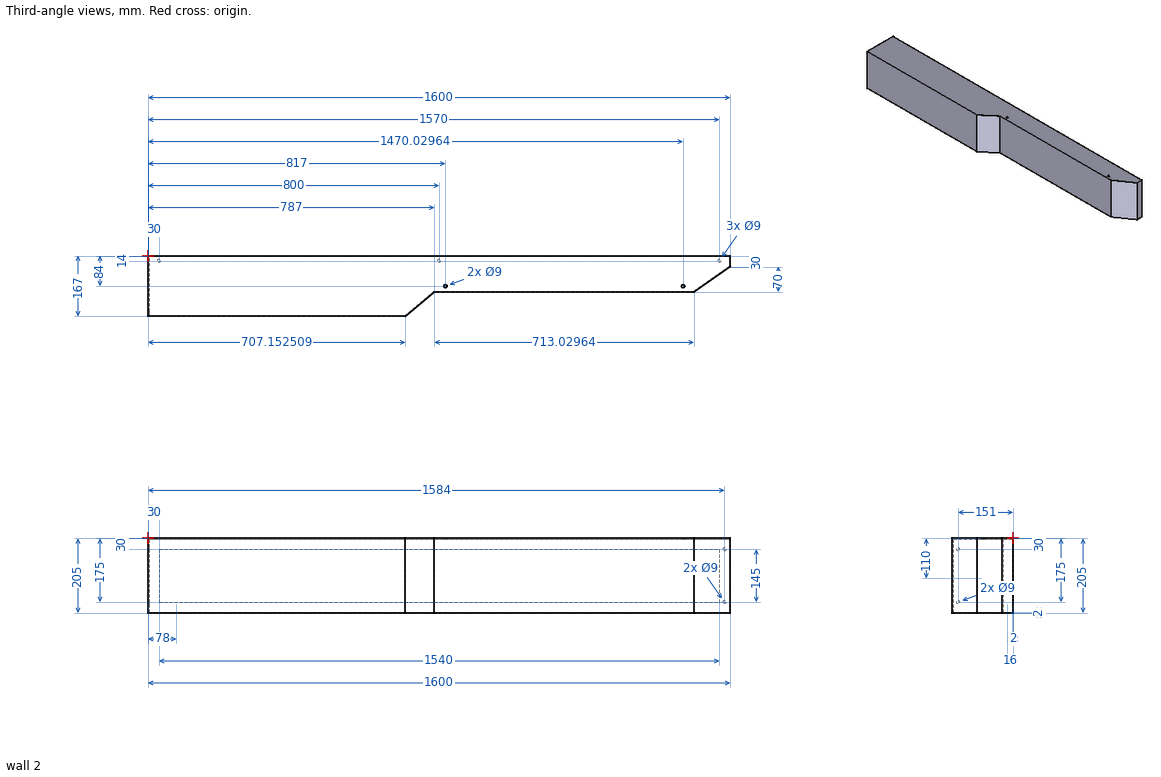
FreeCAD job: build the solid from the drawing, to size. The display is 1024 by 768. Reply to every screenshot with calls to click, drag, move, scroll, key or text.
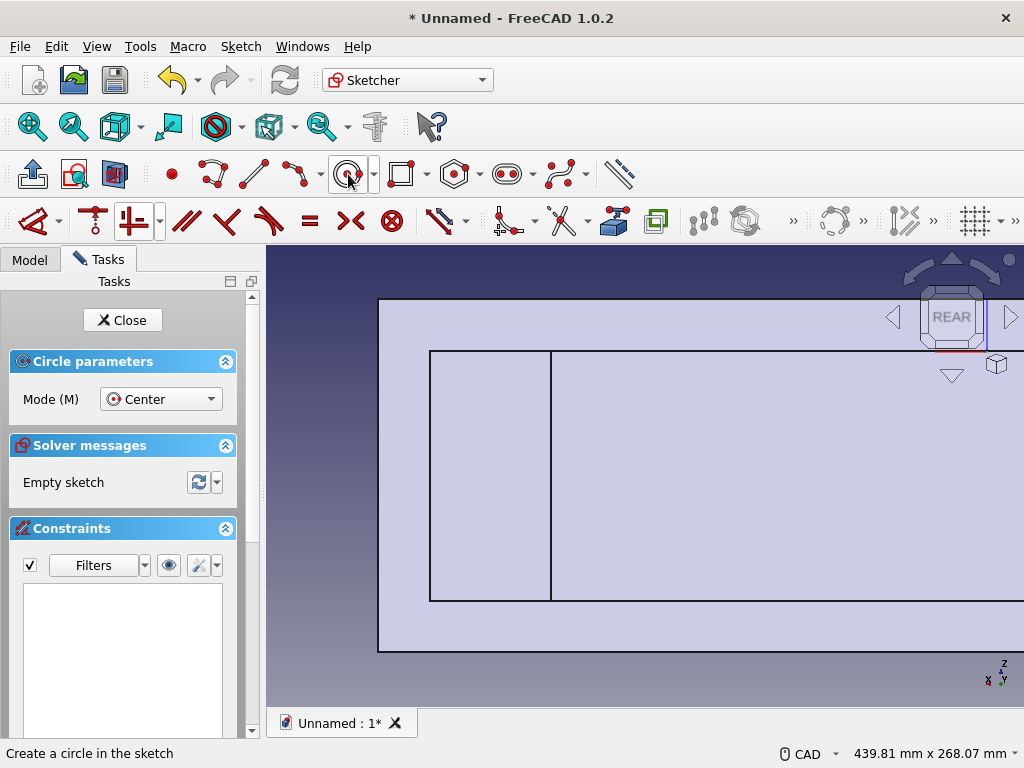
scroll(406, 601, up, 6)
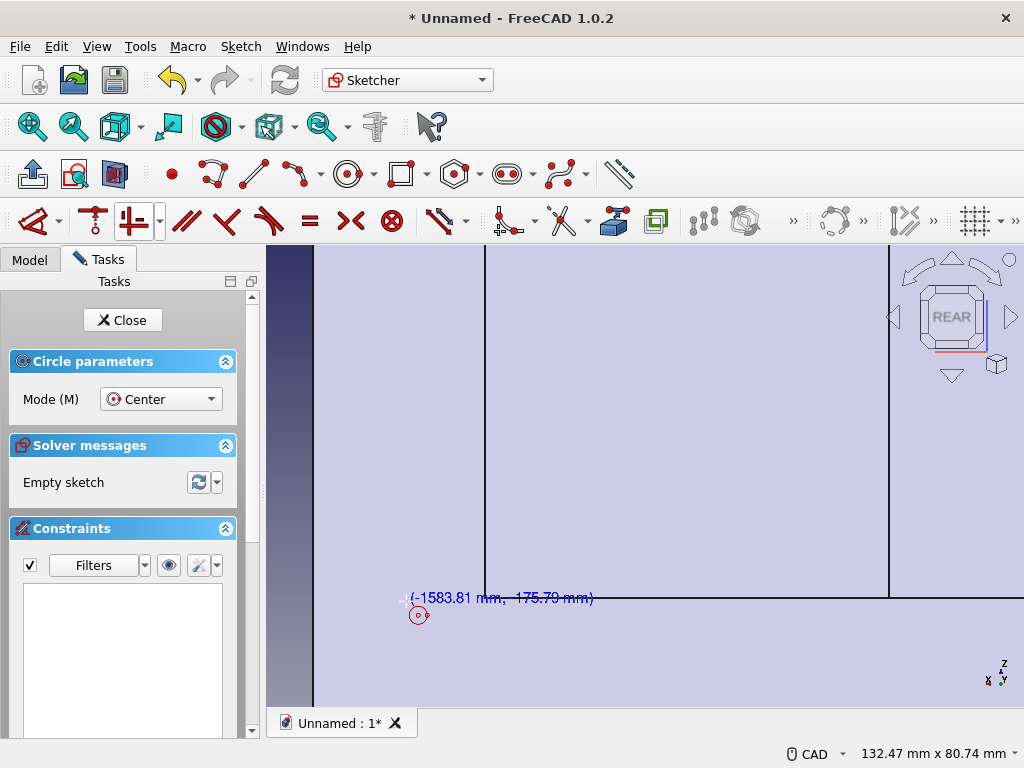
click(405, 598)
move(423, 580)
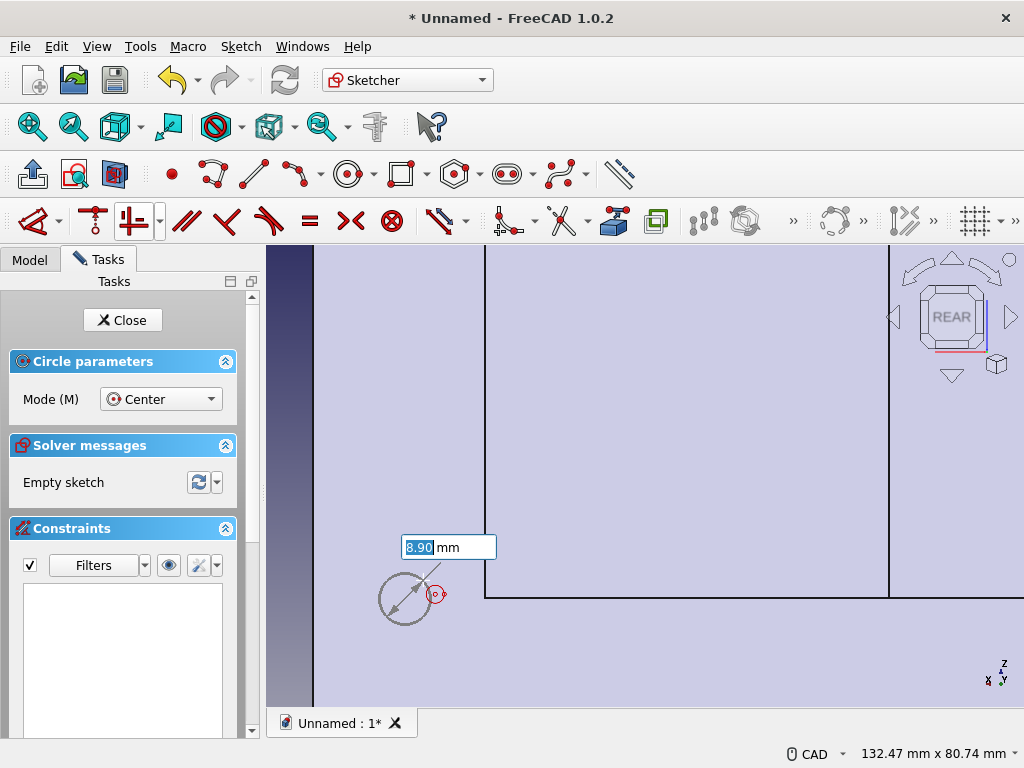
text(9)
key(Return)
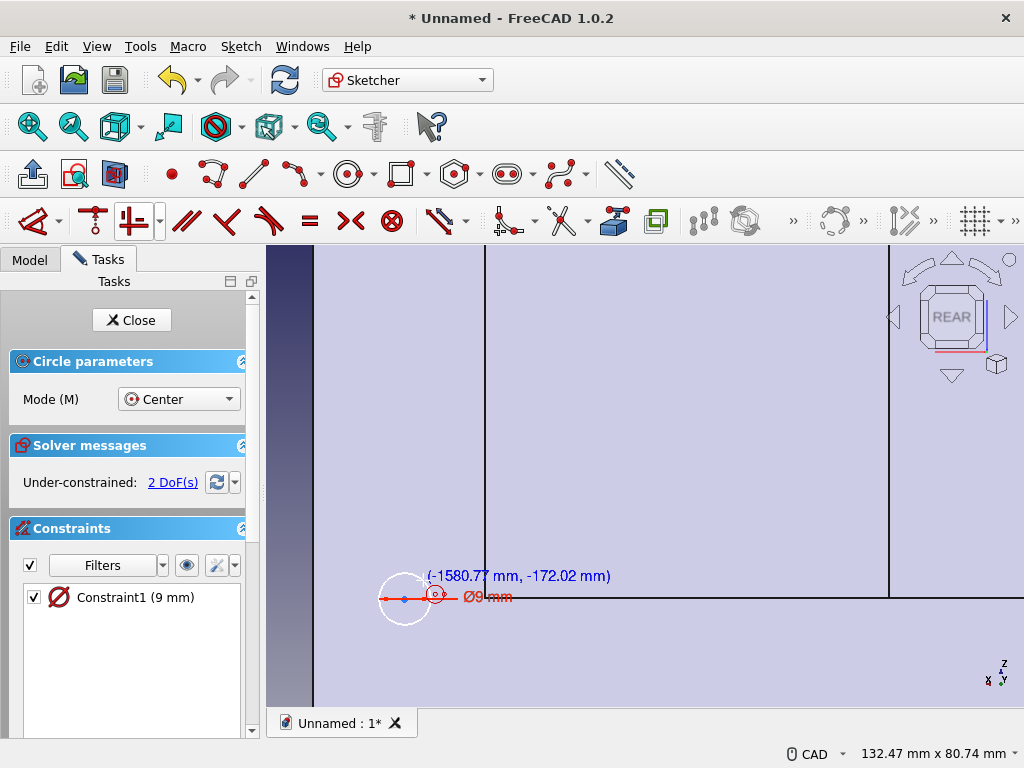
scroll(651, 602, down, 6)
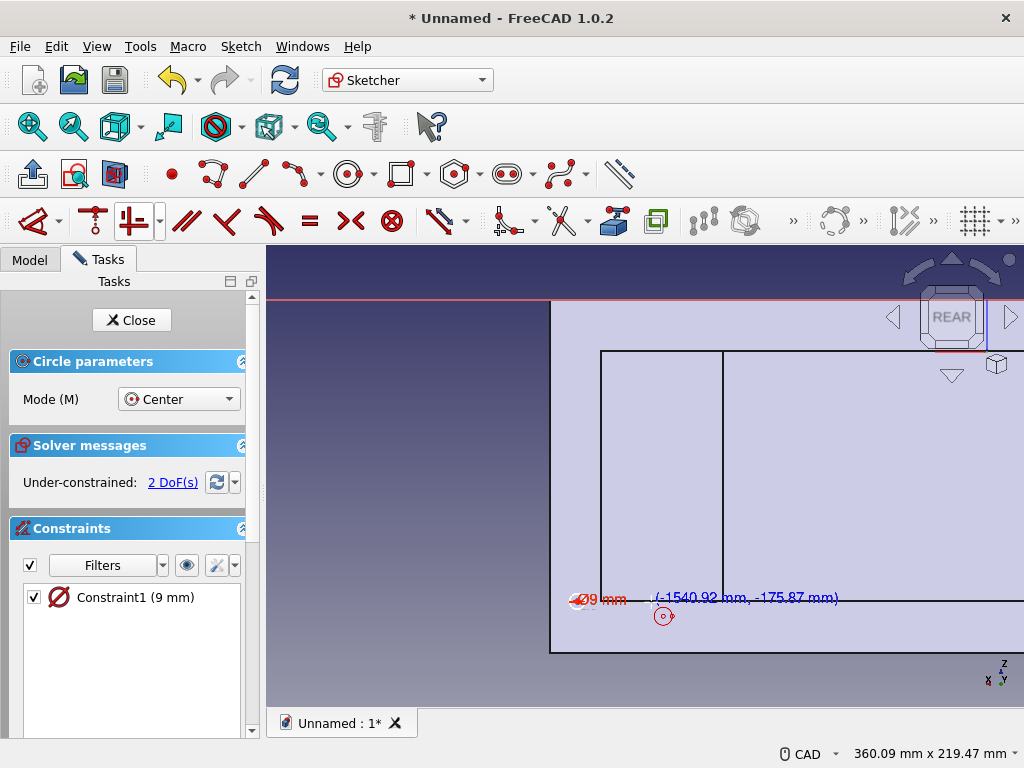
scroll(577, 351, up, 6)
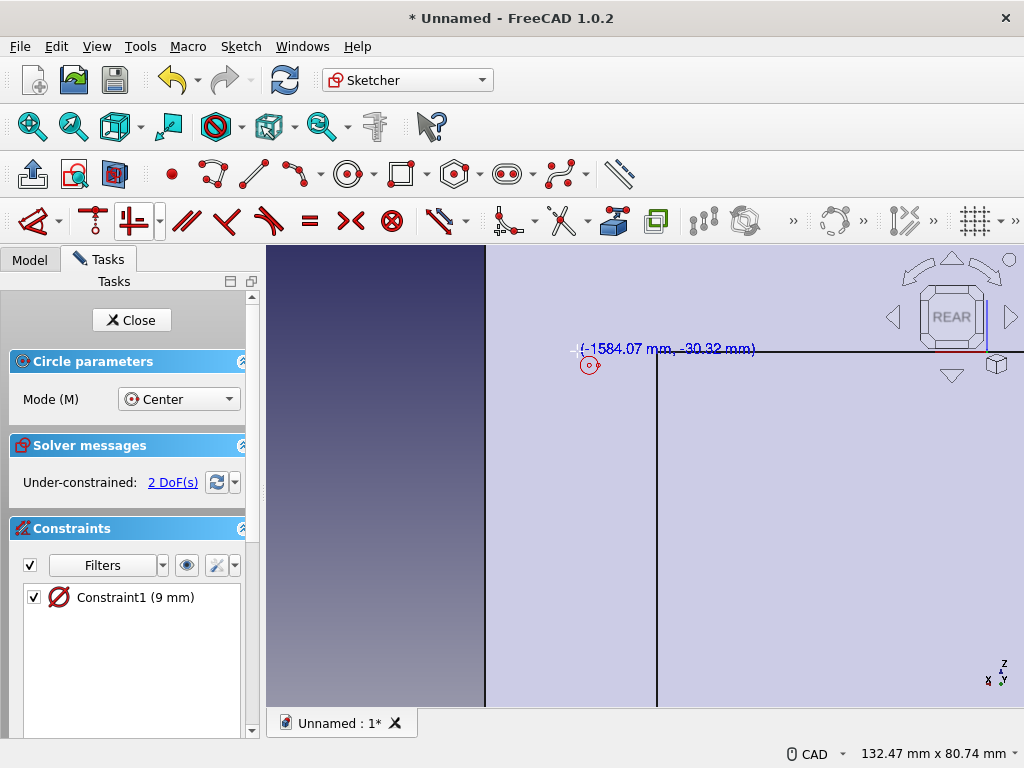
click(576, 352)
move(595, 334)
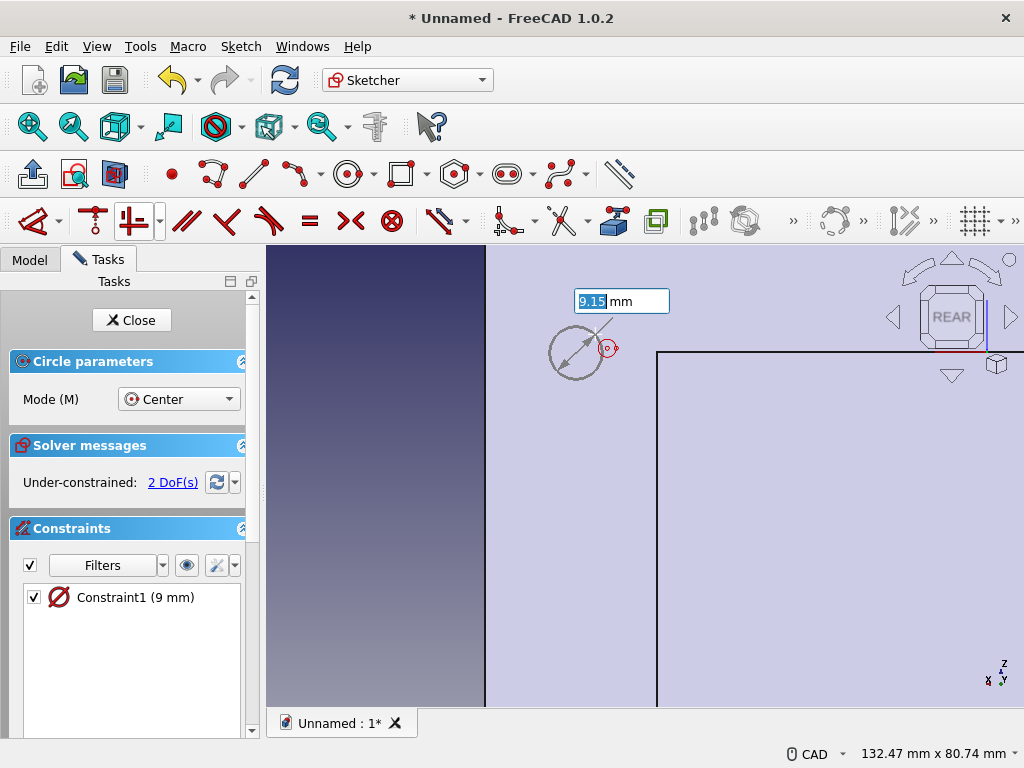
text(9)
key(Return)
key(Escape)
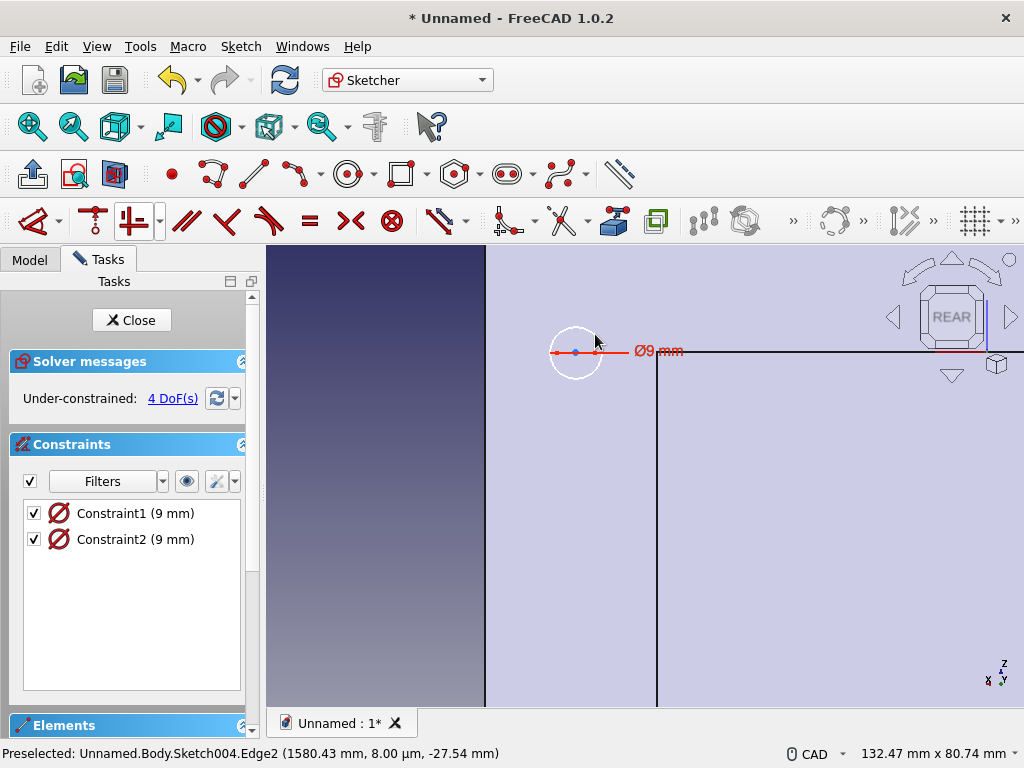
key(d)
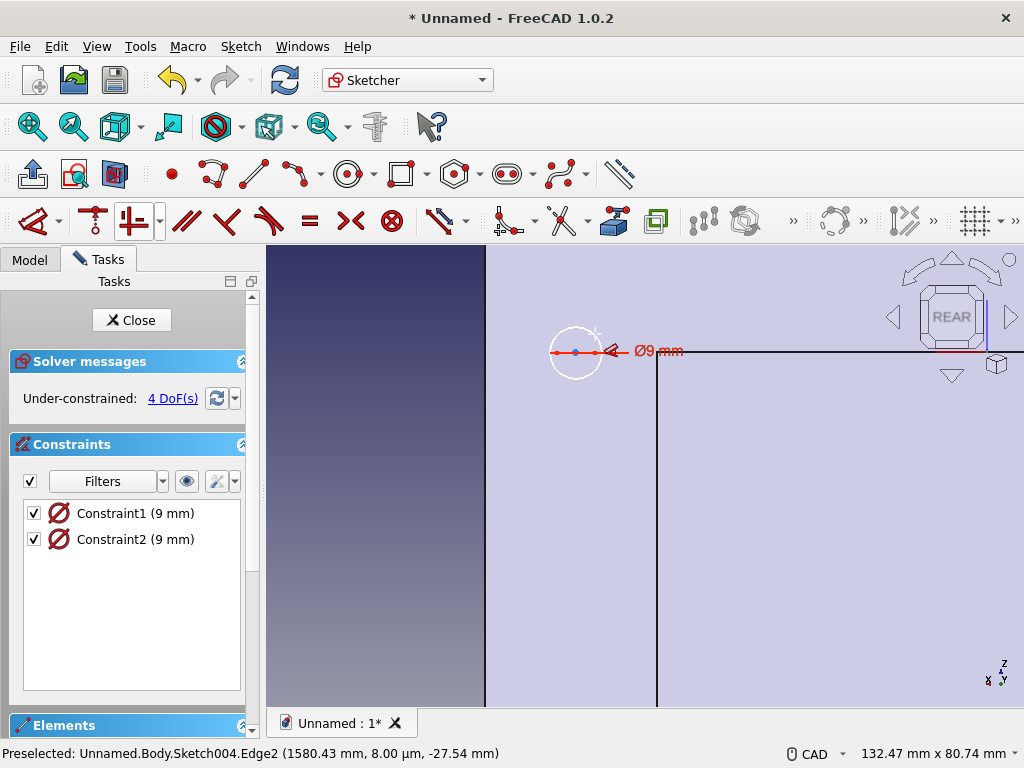
click(576, 353)
click(542, 313)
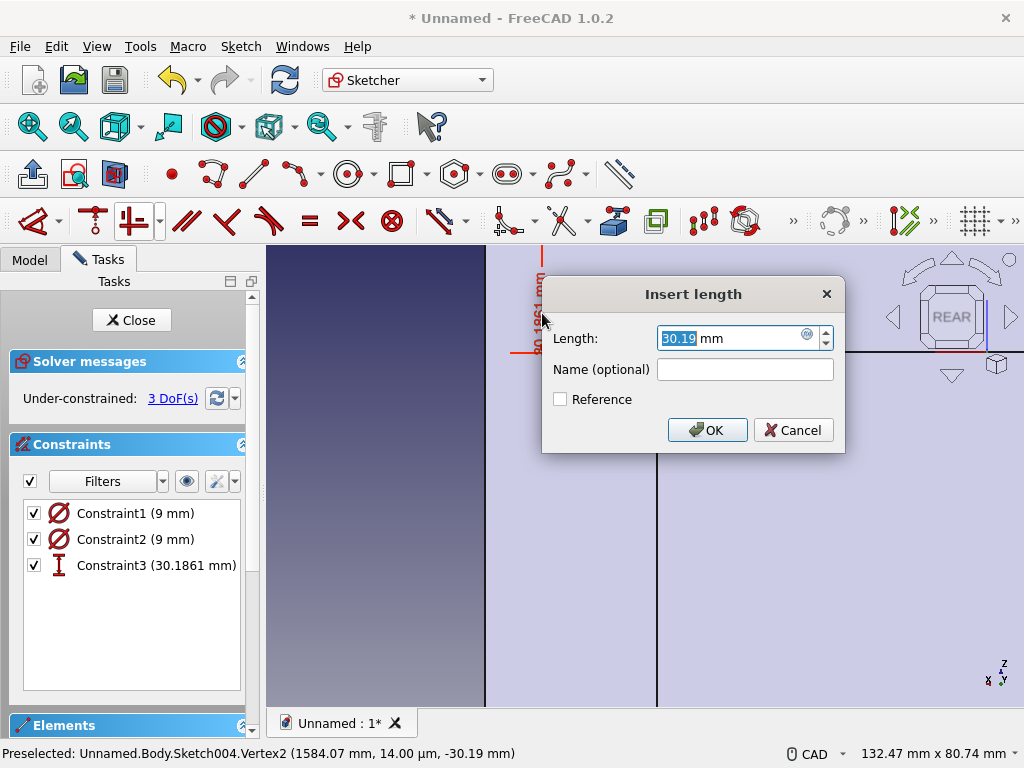
text(30)
key(Return)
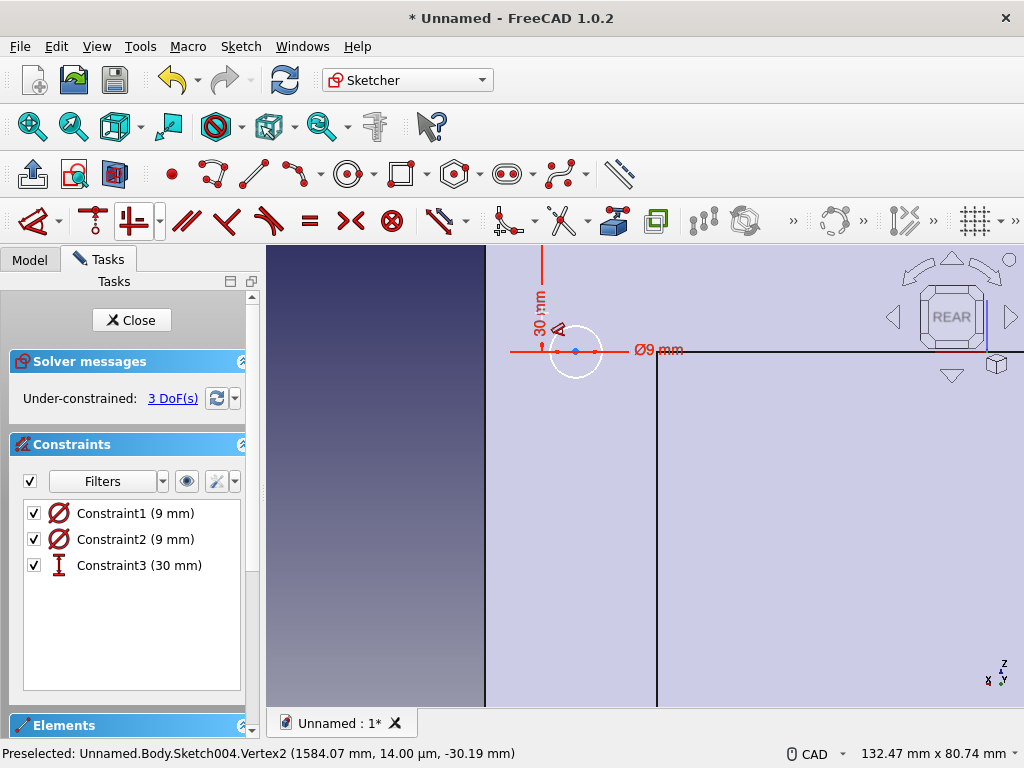
scroll(577, 351, down, 6)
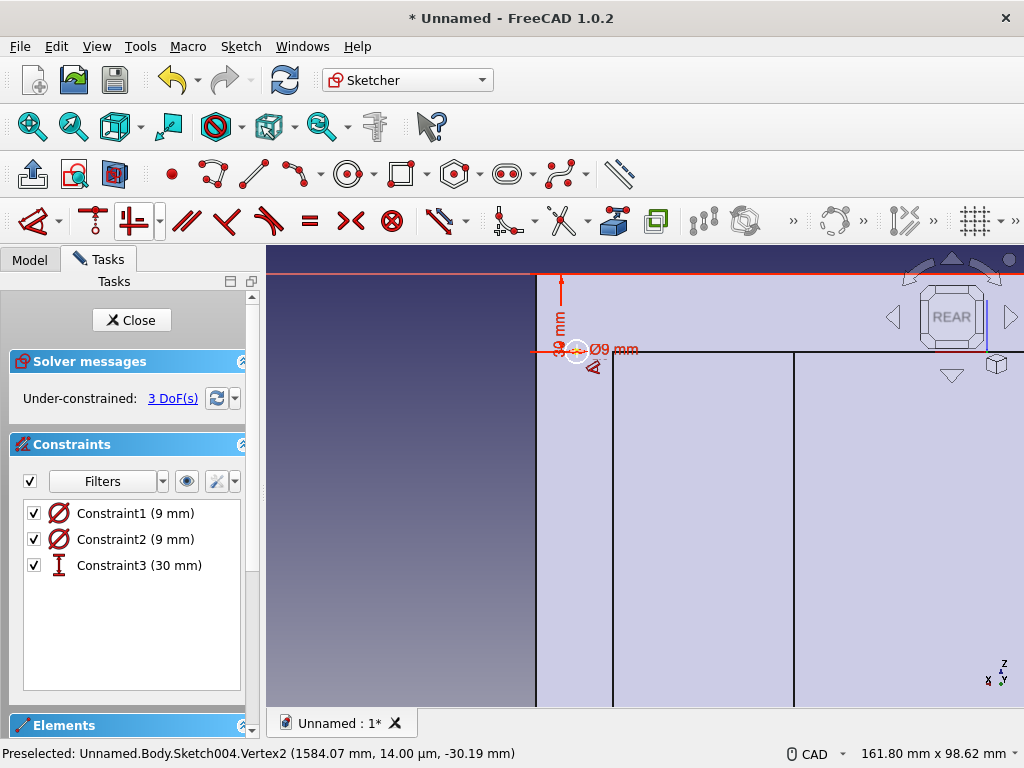
click(577, 602)
click(543, 451)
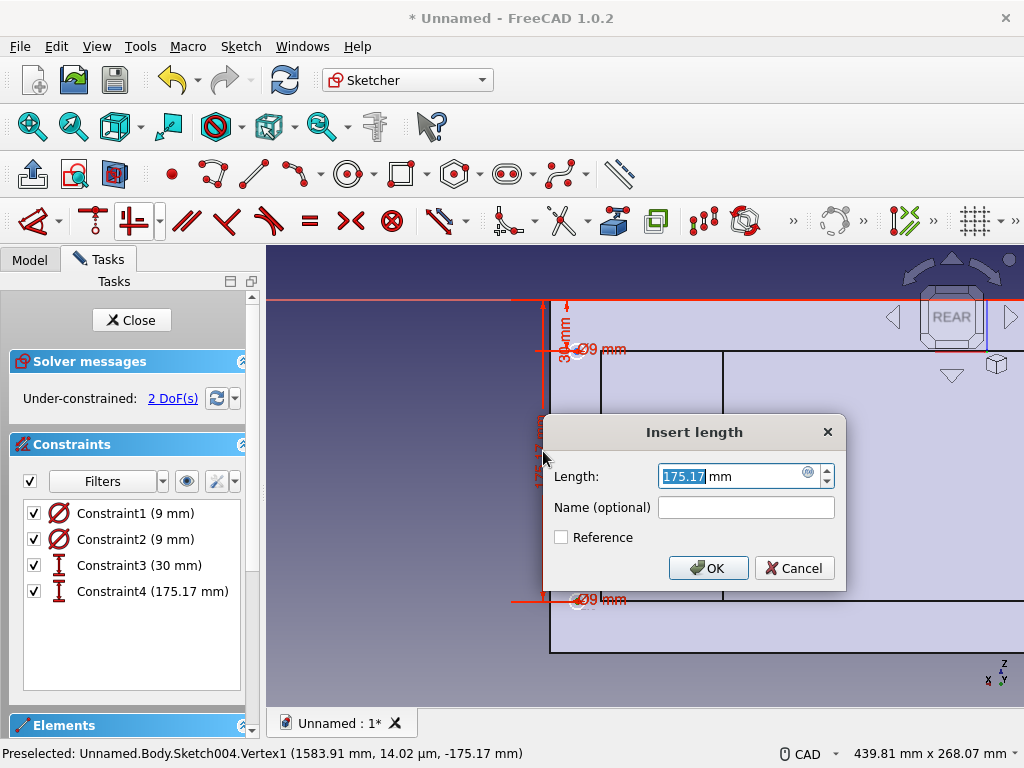
text(175)
key(Return)